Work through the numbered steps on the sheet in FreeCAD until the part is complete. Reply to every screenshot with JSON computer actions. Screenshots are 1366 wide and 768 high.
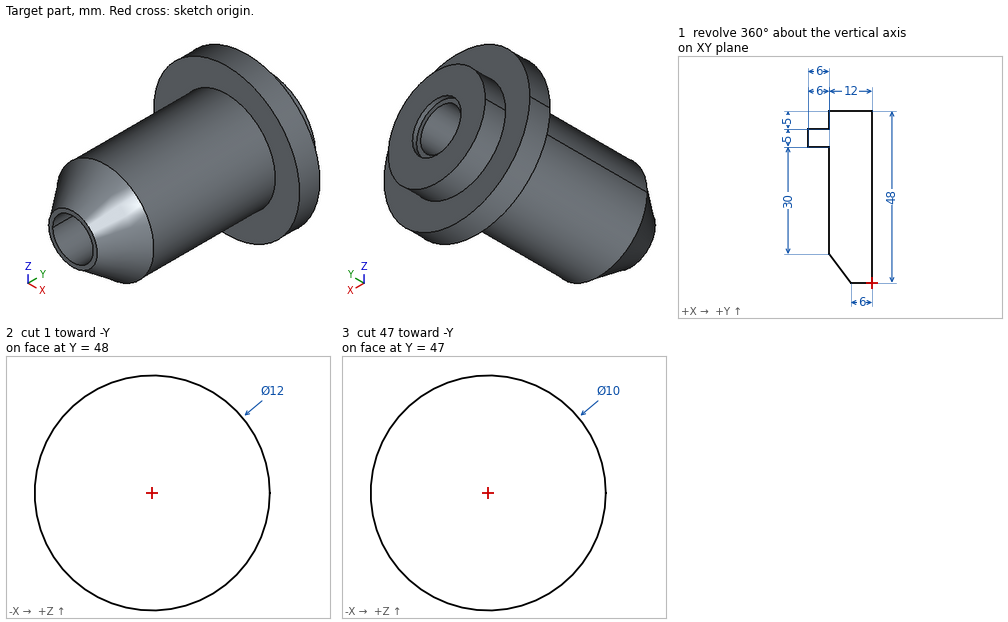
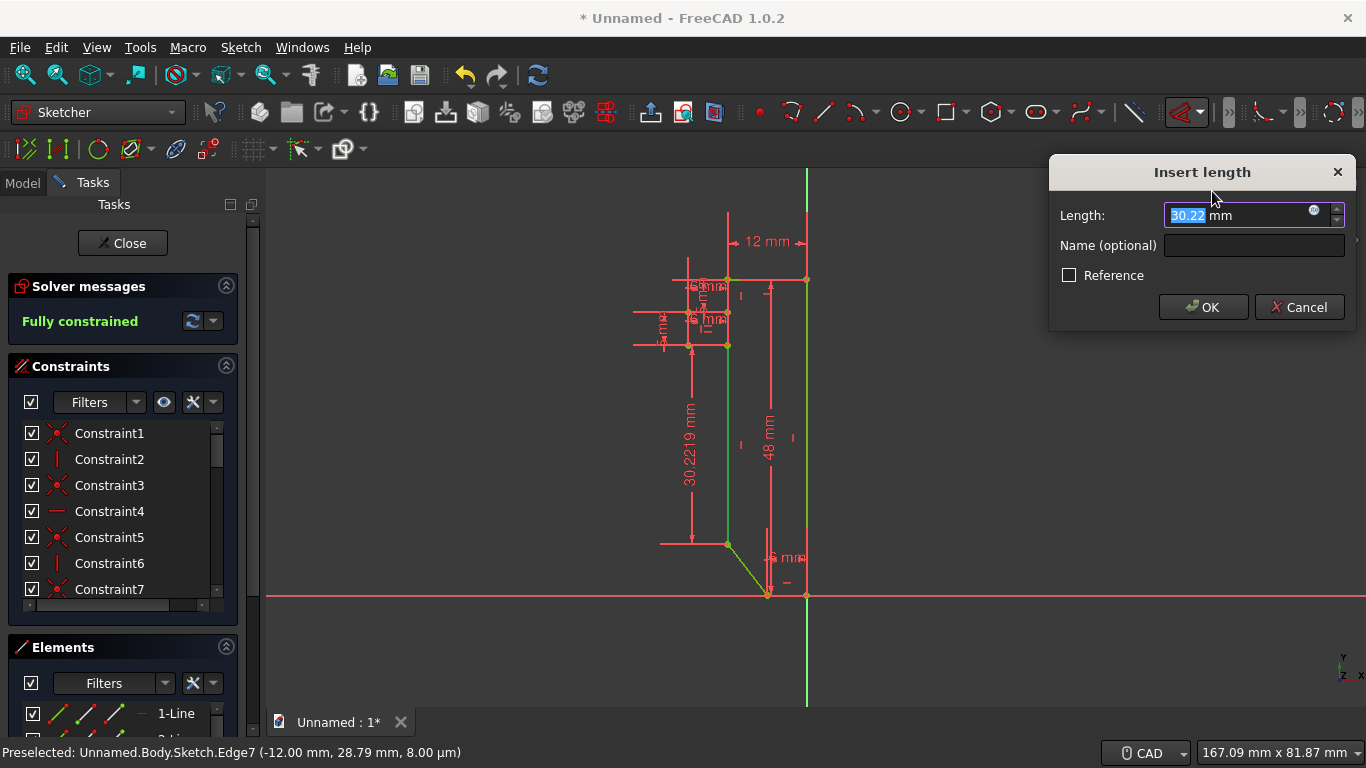
{"action": "type", "text": "30"}
{"action": "key", "text": "Return"}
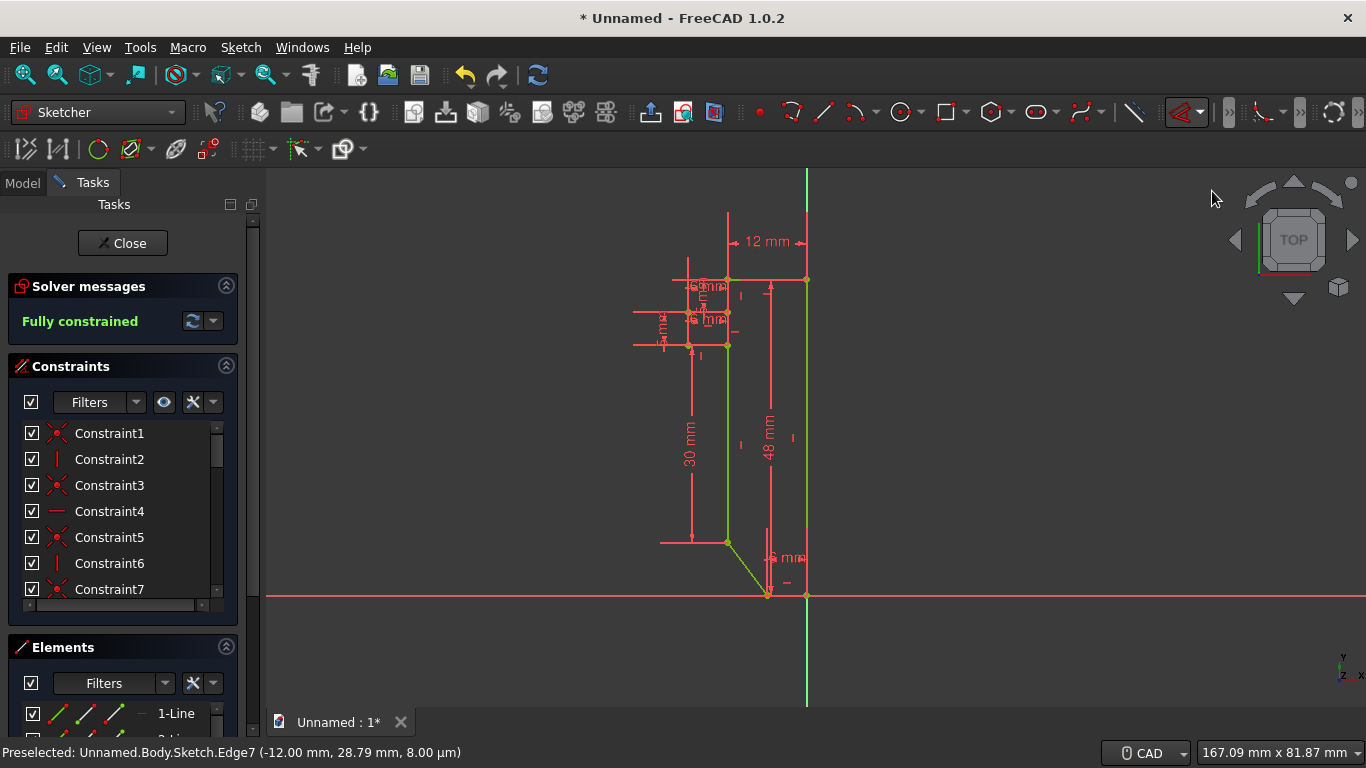
{"action": "left_click", "coordinate": [123, 243]}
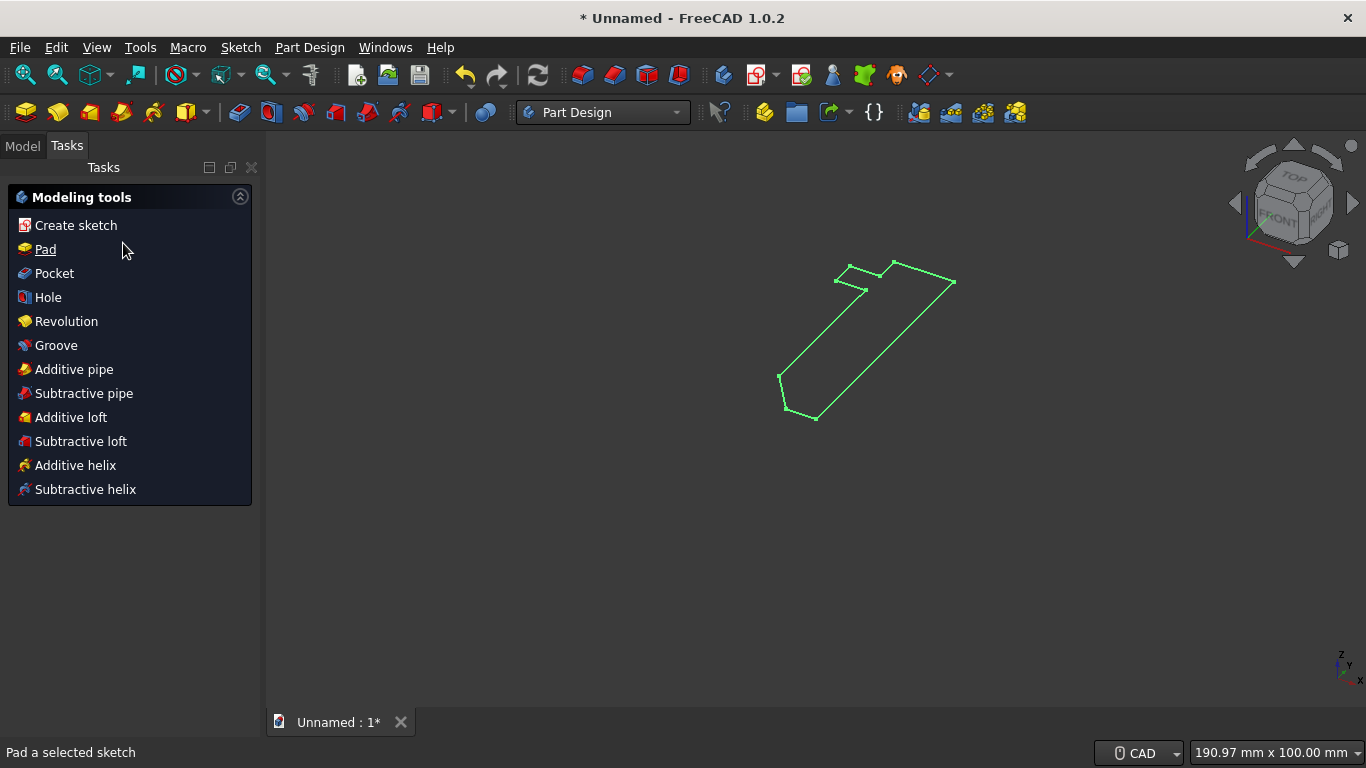
{"action": "left_click", "coordinate": [58, 112]}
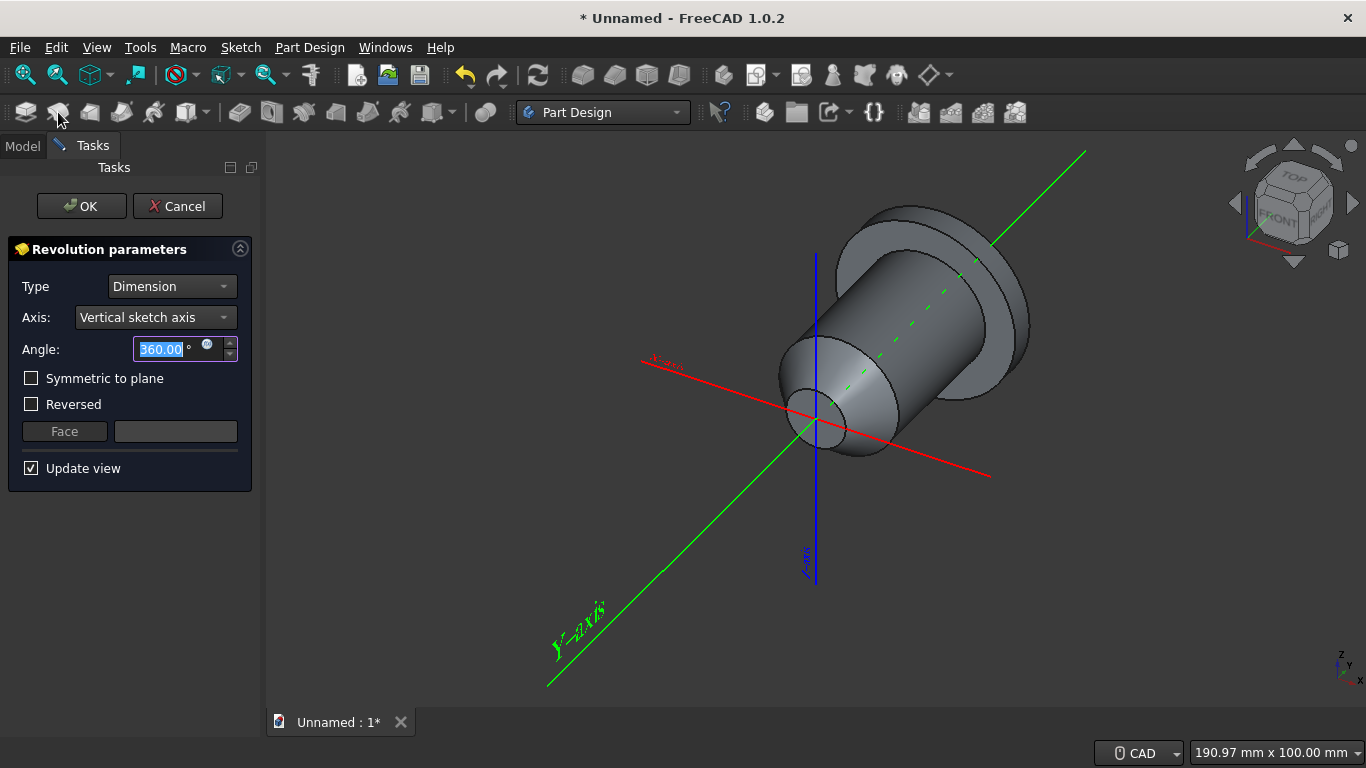
{"action": "left_click", "coordinate": [82, 206]}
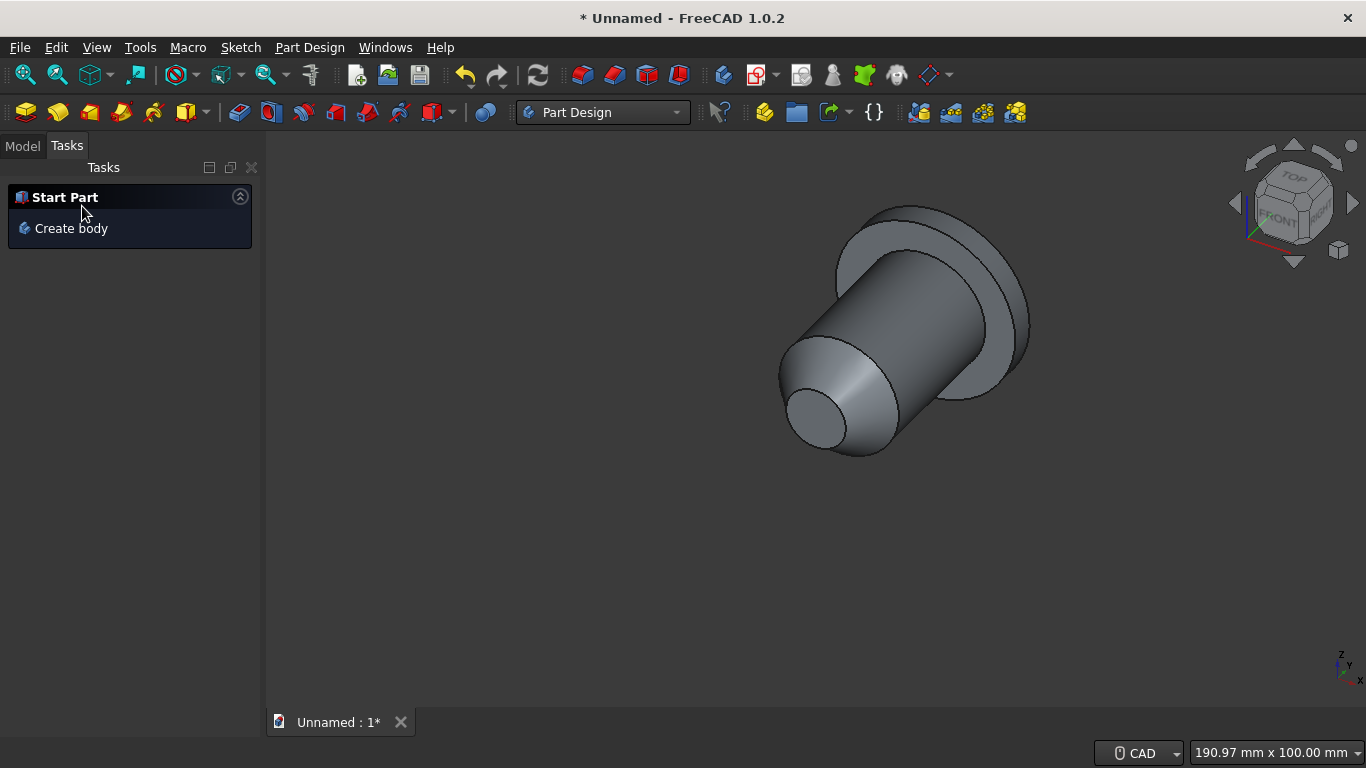
{"action": "key", "text": "4"}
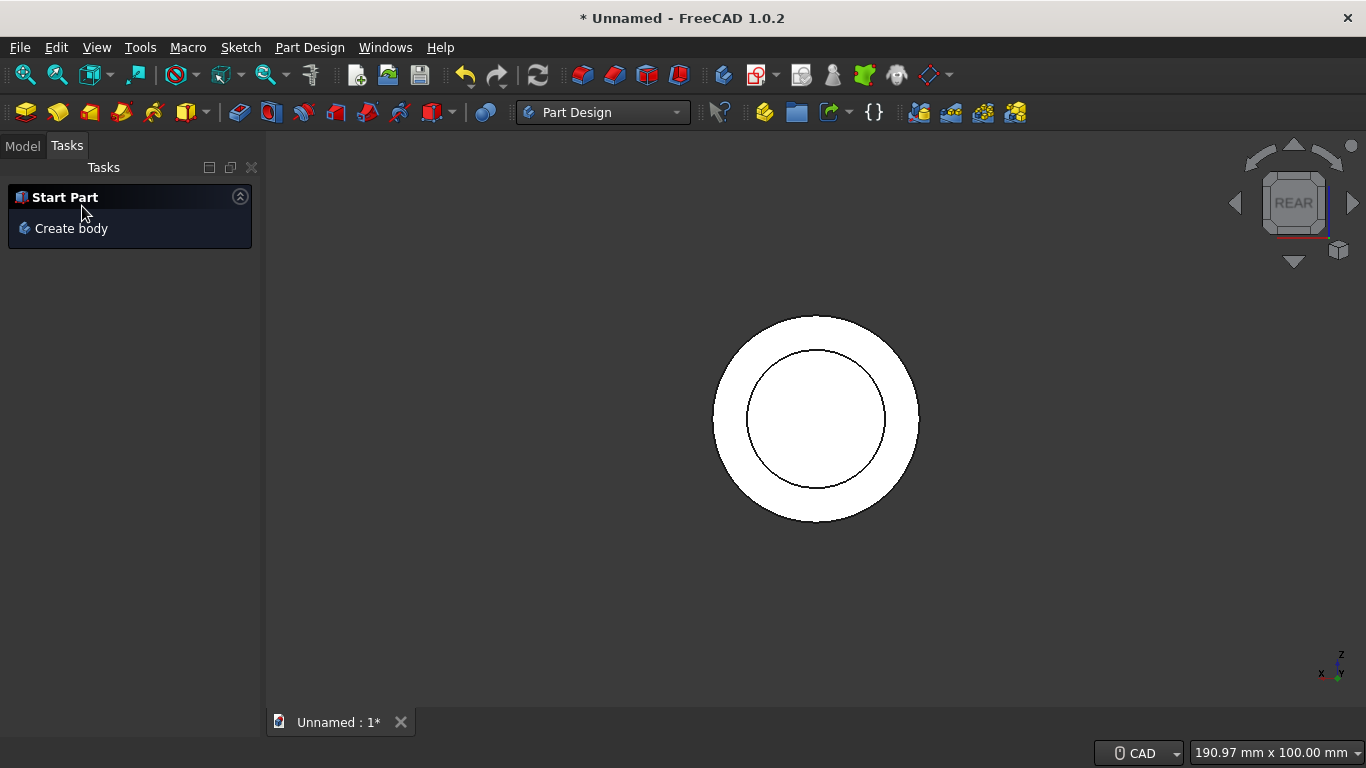
{"action": "left_click", "coordinate": [26, 76]}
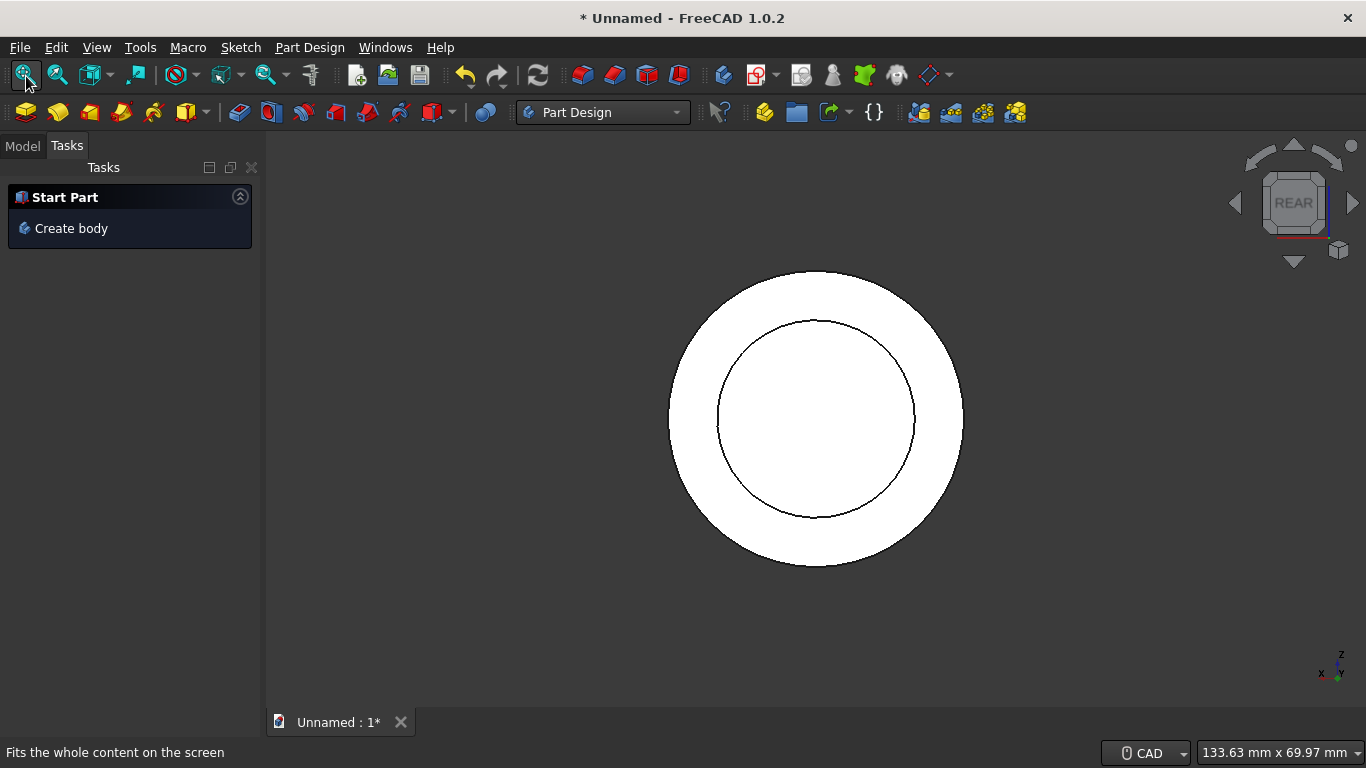
{"action": "left_click", "coordinate": [816, 418]}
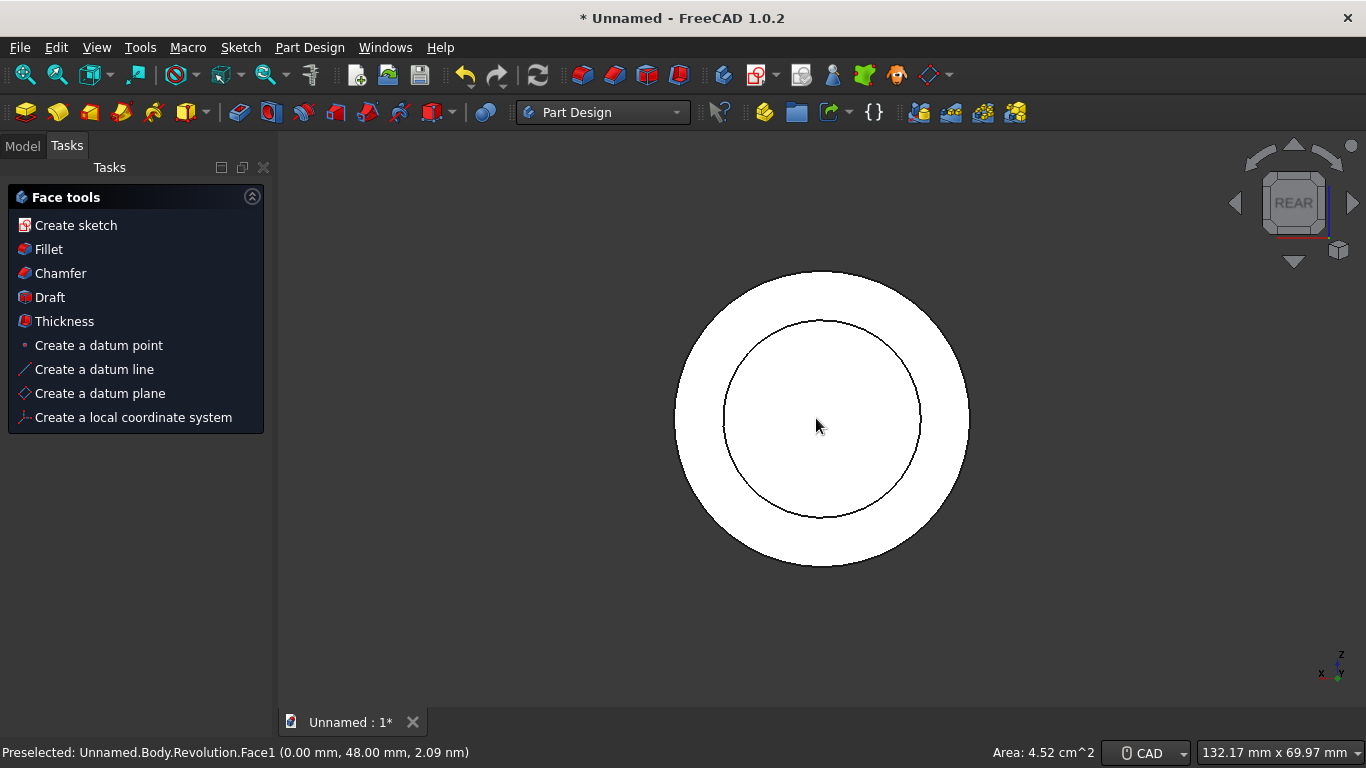
{"action": "left_click", "coordinate": [756, 76]}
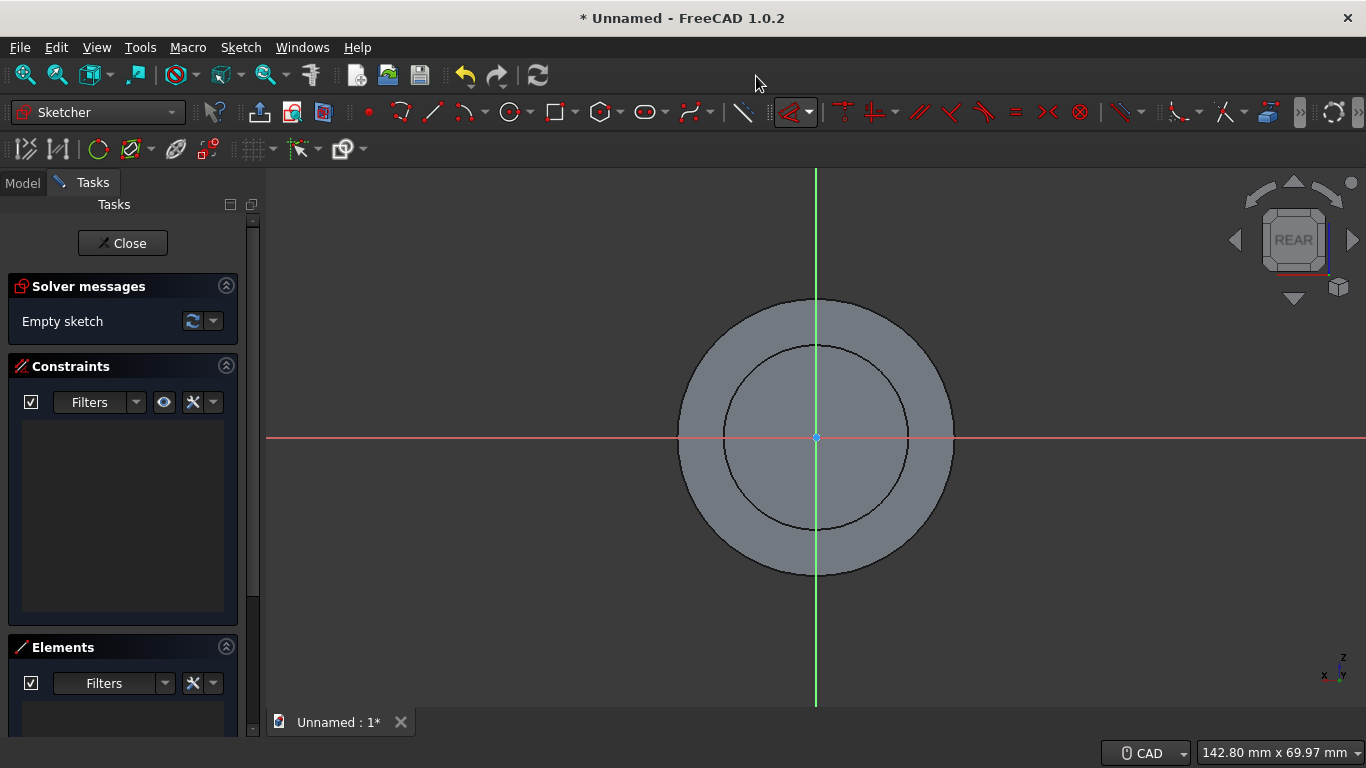
{"action": "scroll", "coordinate": [838, 438], "scroll_direction": "up", "scroll_amount": 7}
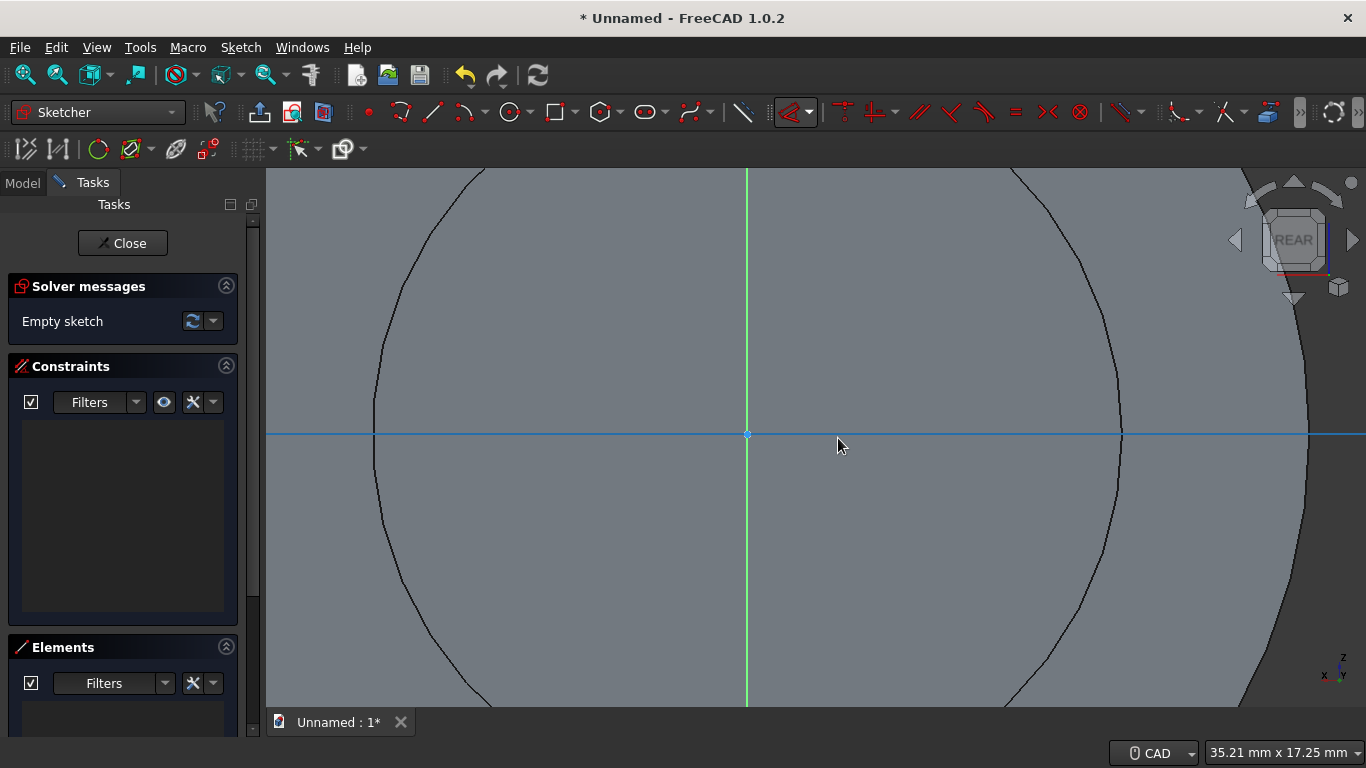
{"action": "left_click", "coordinate": [510, 112]}